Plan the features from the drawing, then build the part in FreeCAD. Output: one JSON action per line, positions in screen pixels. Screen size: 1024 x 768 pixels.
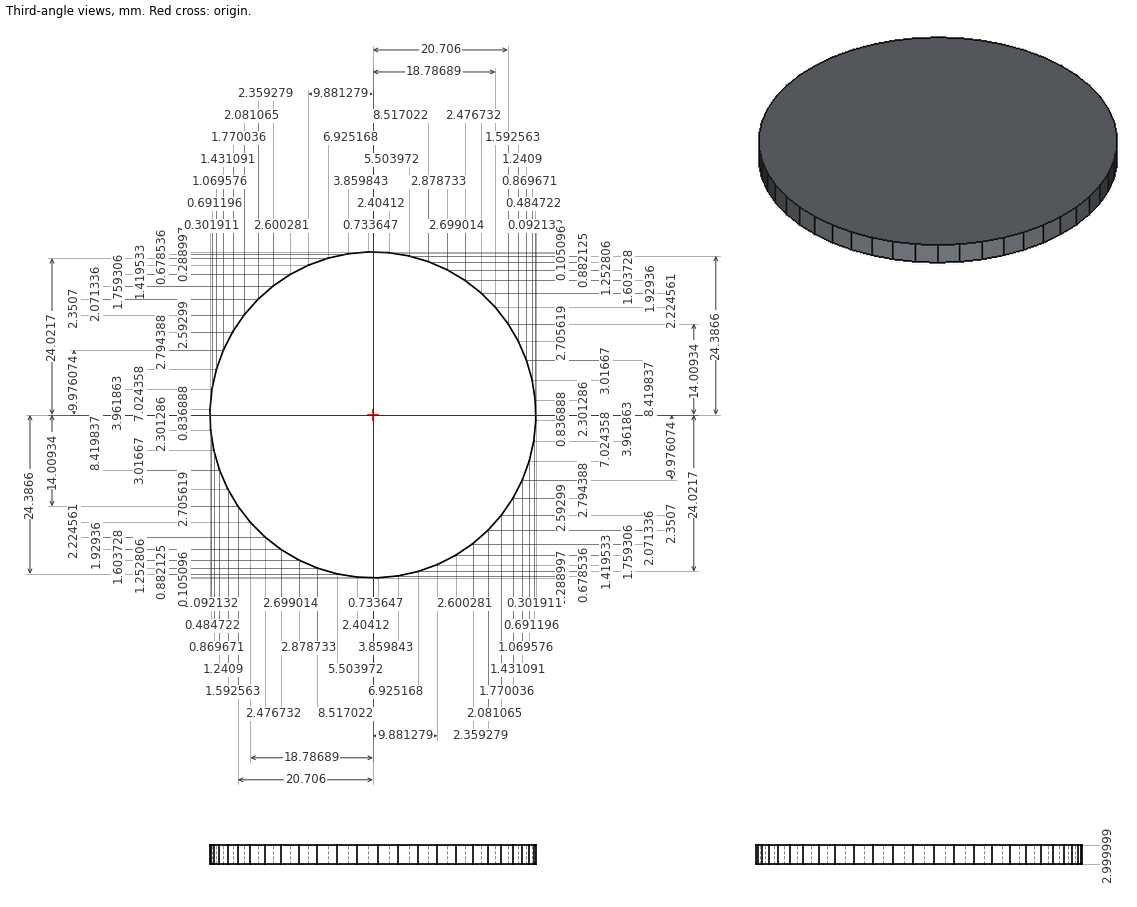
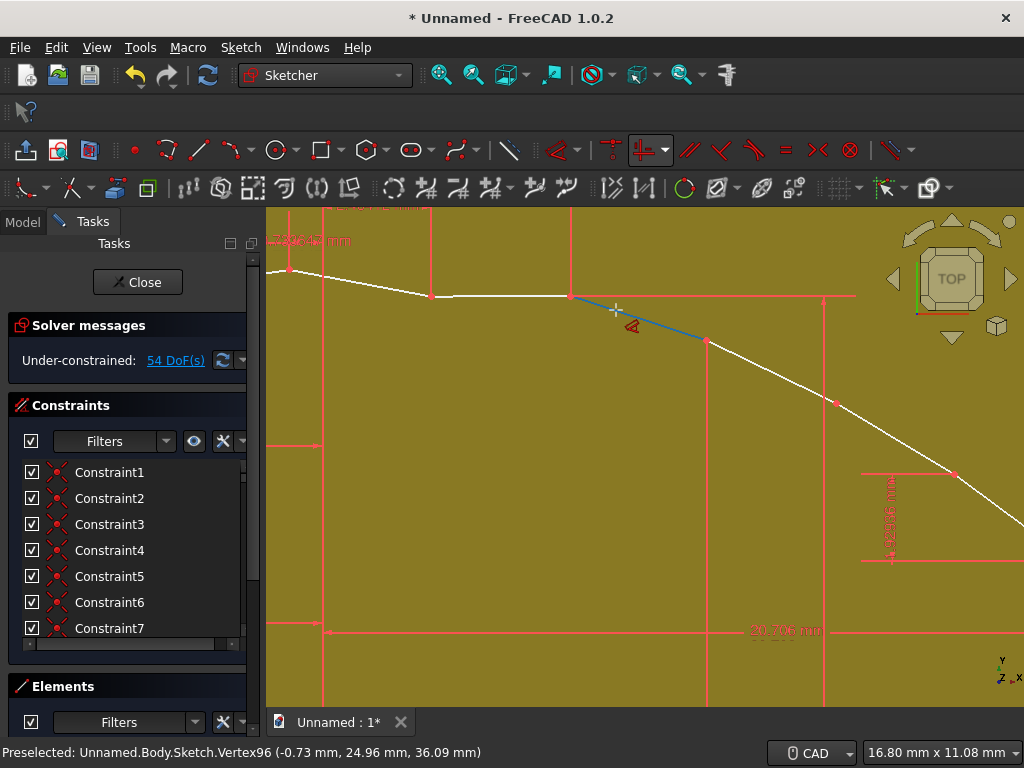
{"action": "left_click", "coordinate": [612, 309]}
{"action": "left_click", "coordinate": [741, 318]}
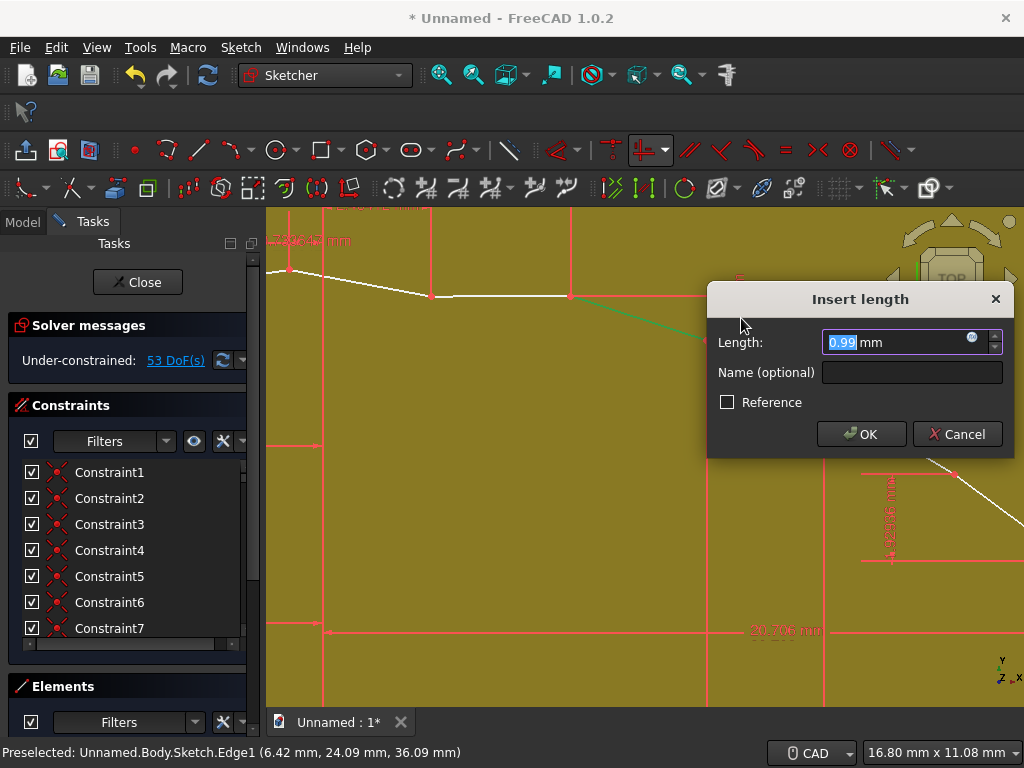
{"action": "type", "text": "0.882125"}
{"action": "key", "text": "Return"}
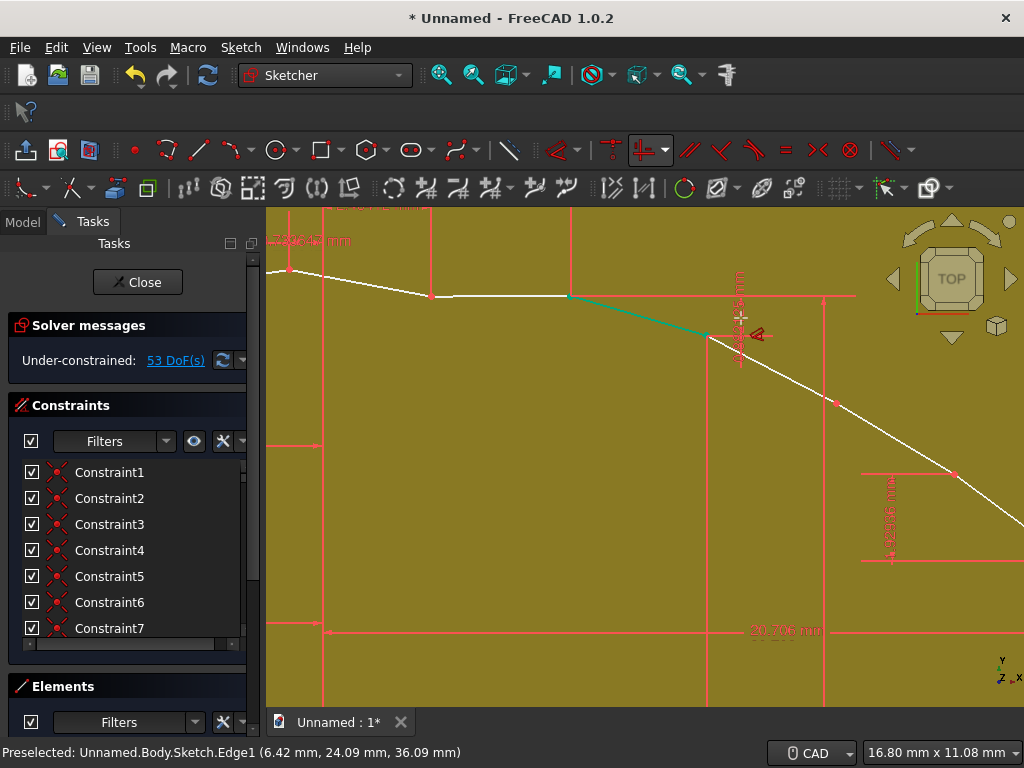
{"action": "scroll", "coordinate": [616, 310], "scroll_direction": "down", "scroll_amount": 10}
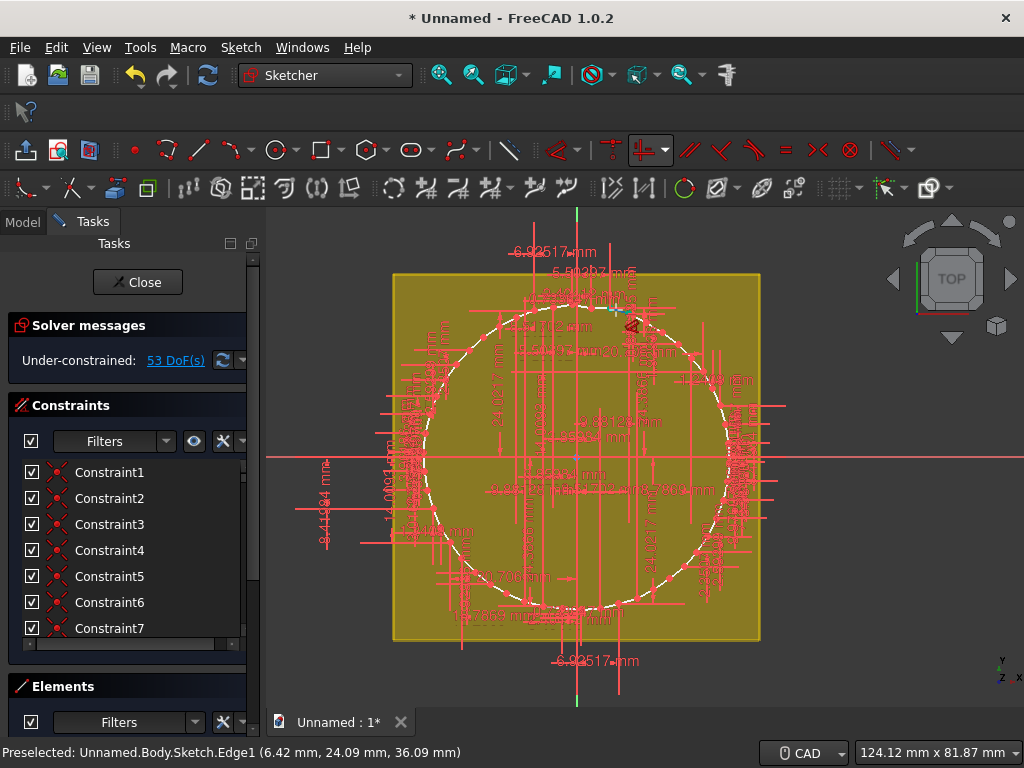
{"action": "scroll", "coordinate": [634, 316], "scroll_direction": "up", "scroll_amount": 5}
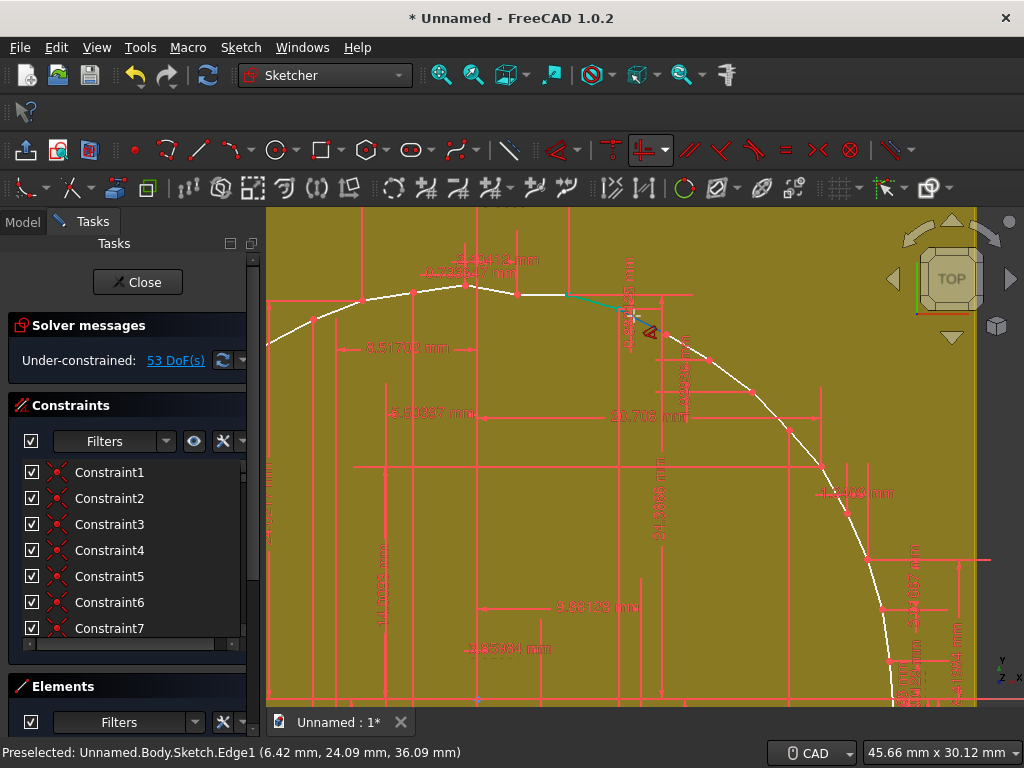
{"action": "left_click", "coordinate": [633, 317]}
{"action": "left_click", "coordinate": [643, 275]}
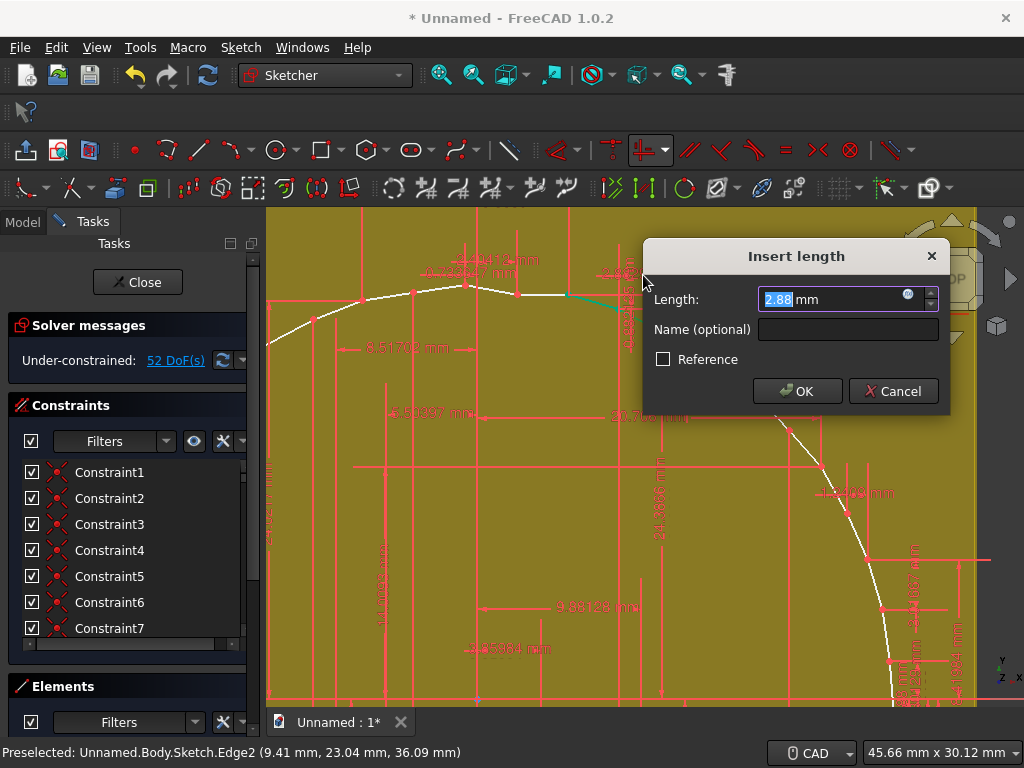
{"action": "type", "text": "2.878733"}
{"action": "key", "text": "Return"}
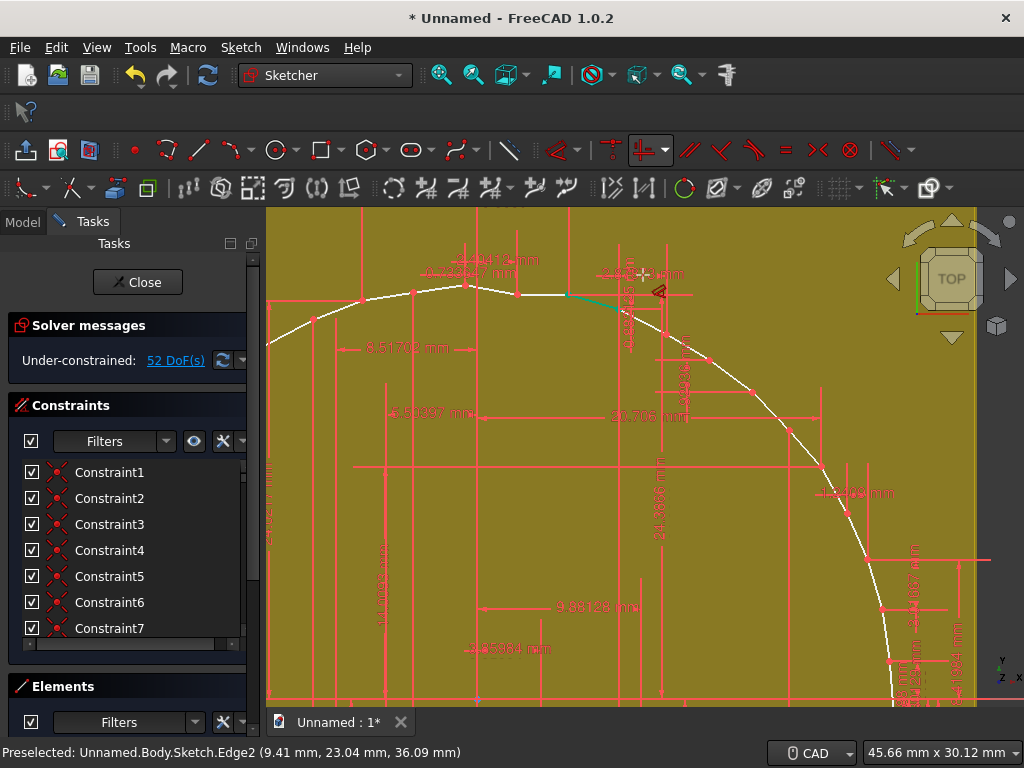
{"action": "scroll", "coordinate": [633, 317], "scroll_direction": "up", "scroll_amount": 4}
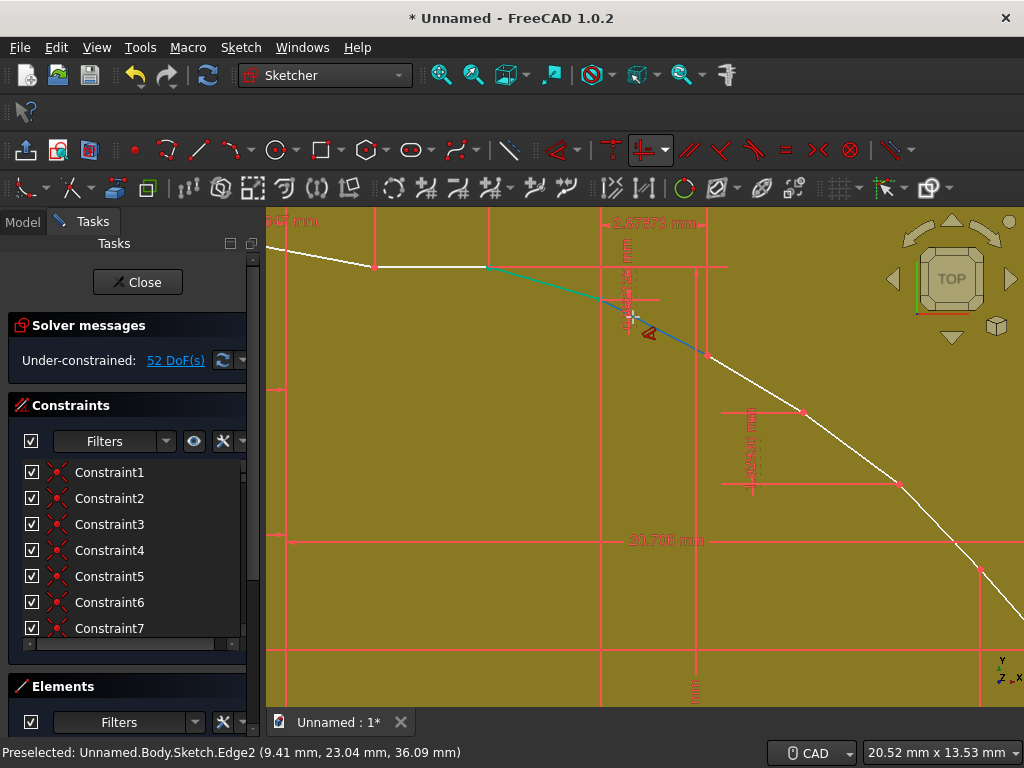
{"action": "left_click", "coordinate": [633, 316]}
{"action": "left_click", "coordinate": [741, 327]}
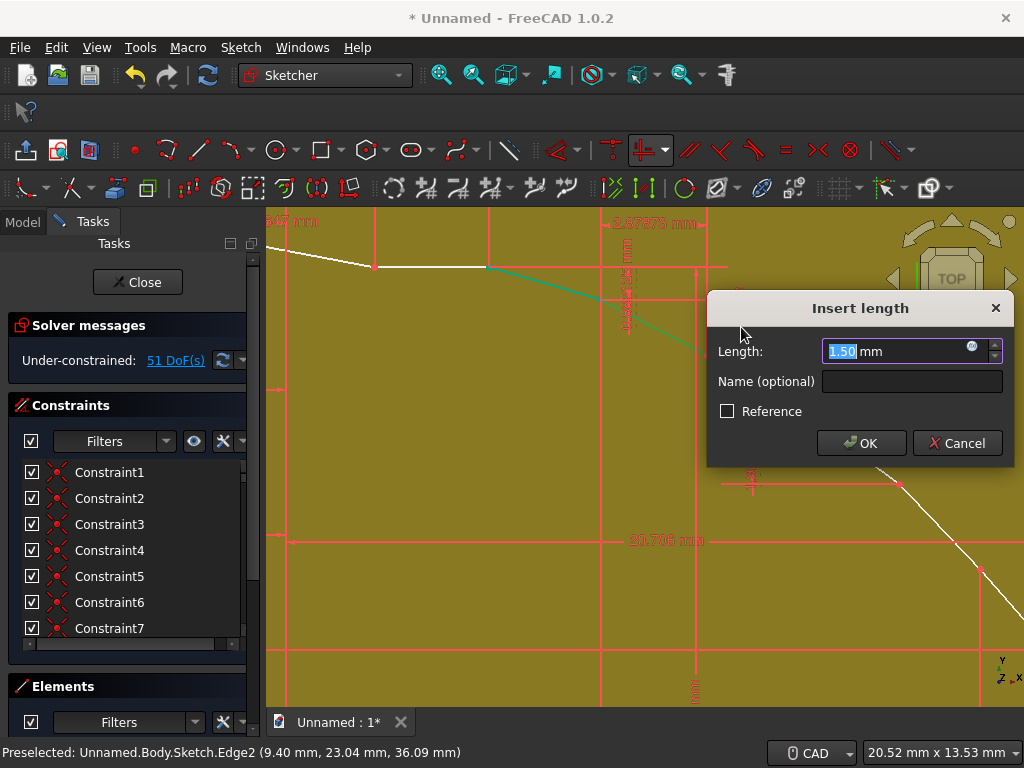
{"action": "type", "text": "1.252806"}
{"action": "key", "text": "Return"}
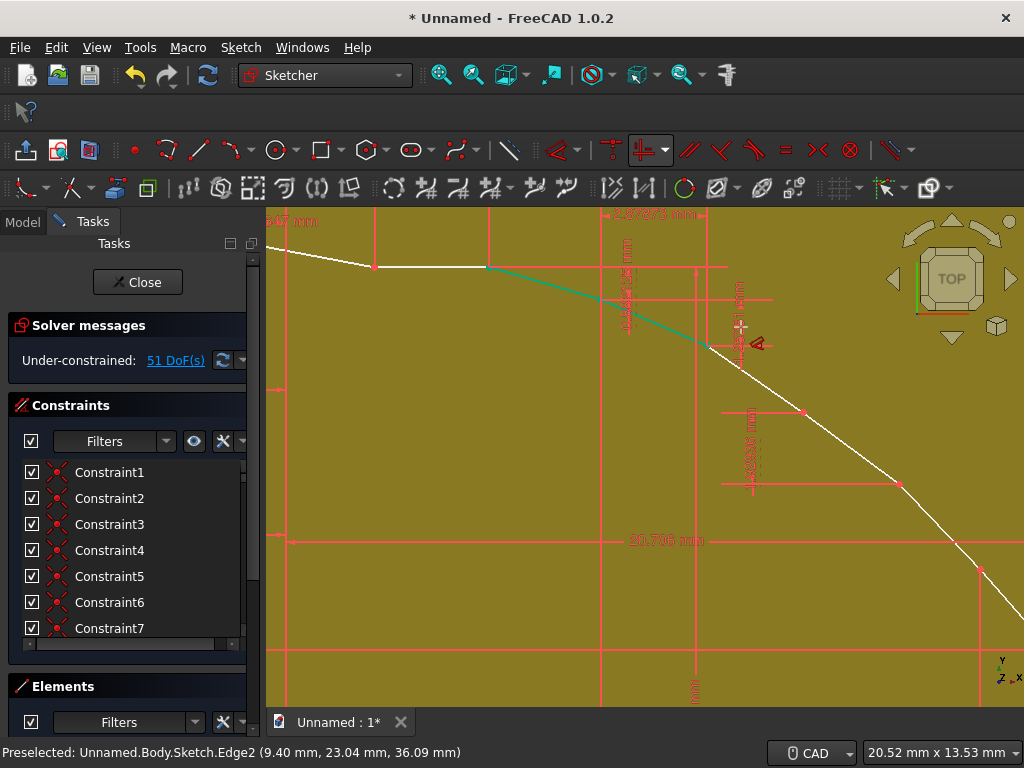
{"action": "left_click", "coordinate": [736, 366]}
{"action": "left_click", "coordinate": [755, 288]}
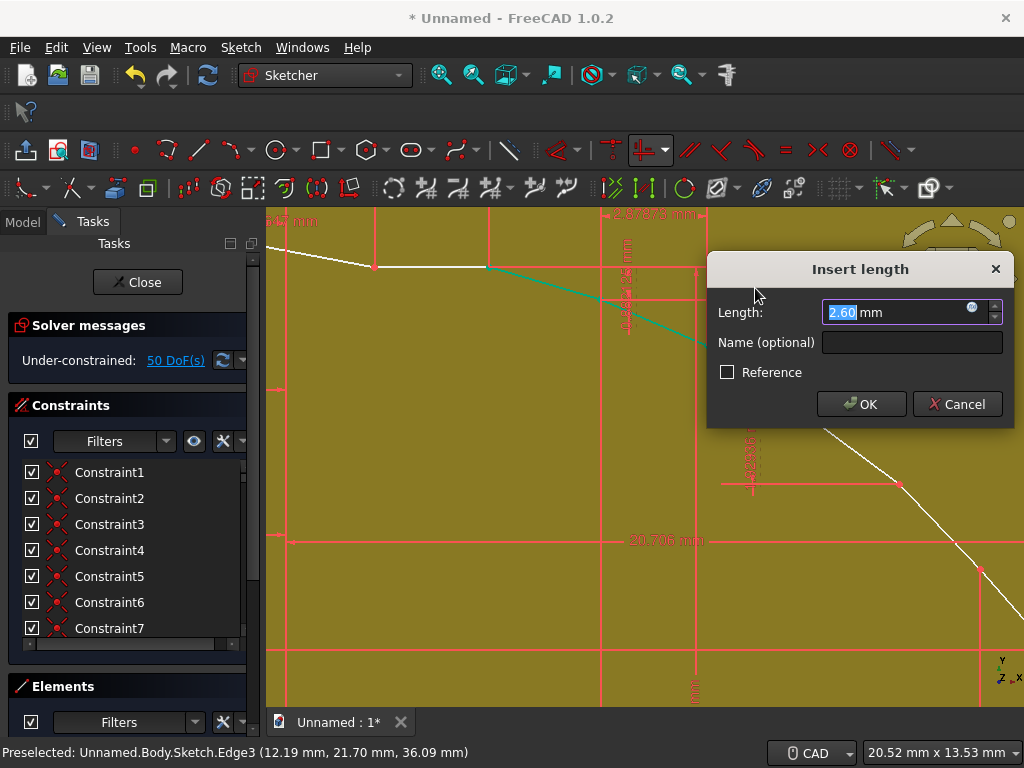
{"action": "type", "text": "2.699014"}
{"action": "key", "text": "Return"}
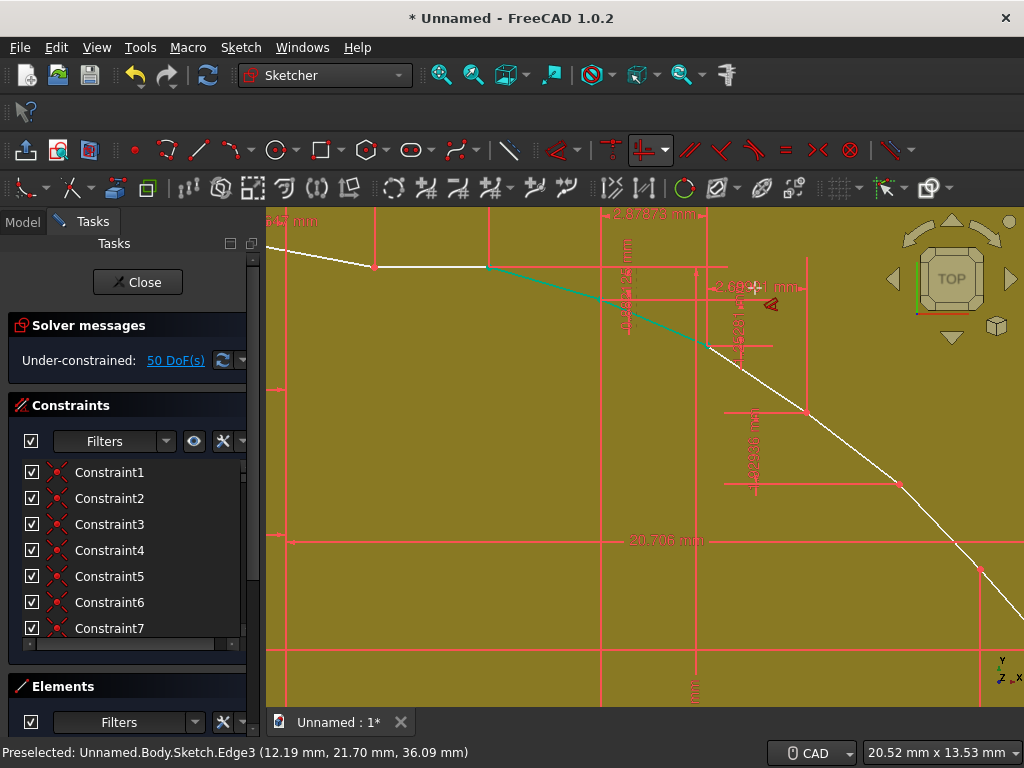
{"action": "left_click", "coordinate": [737, 366]}
{"action": "left_click", "coordinate": [841, 379]}